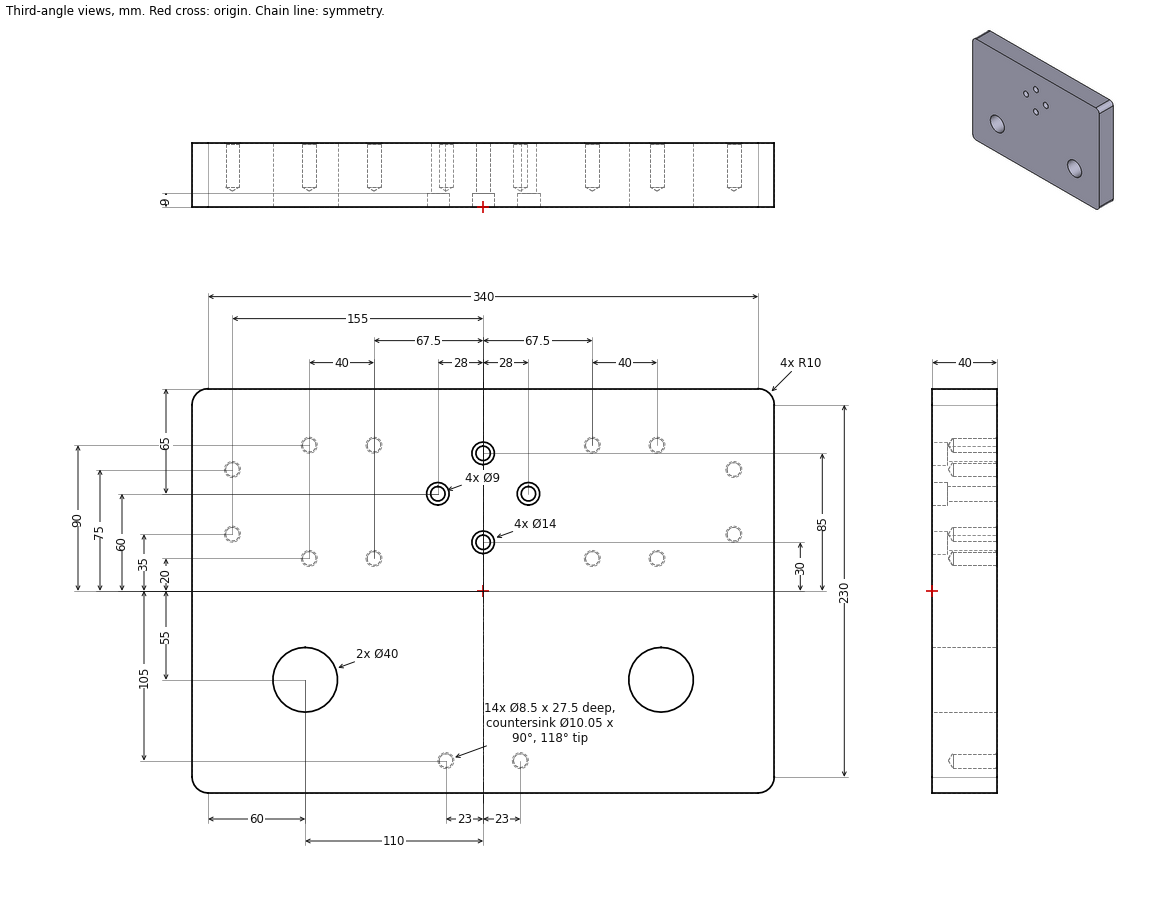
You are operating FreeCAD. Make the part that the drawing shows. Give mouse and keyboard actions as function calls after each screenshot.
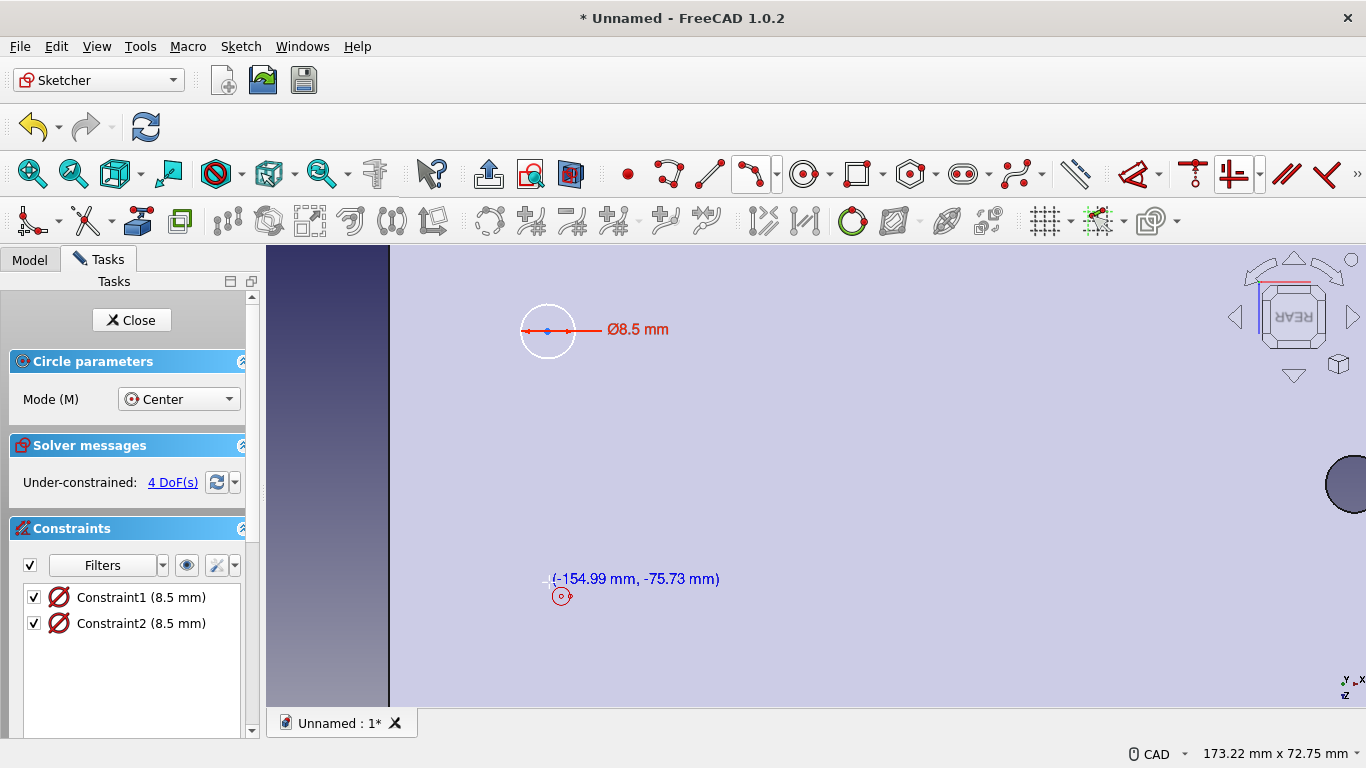
scroll(549, 582, down, 8)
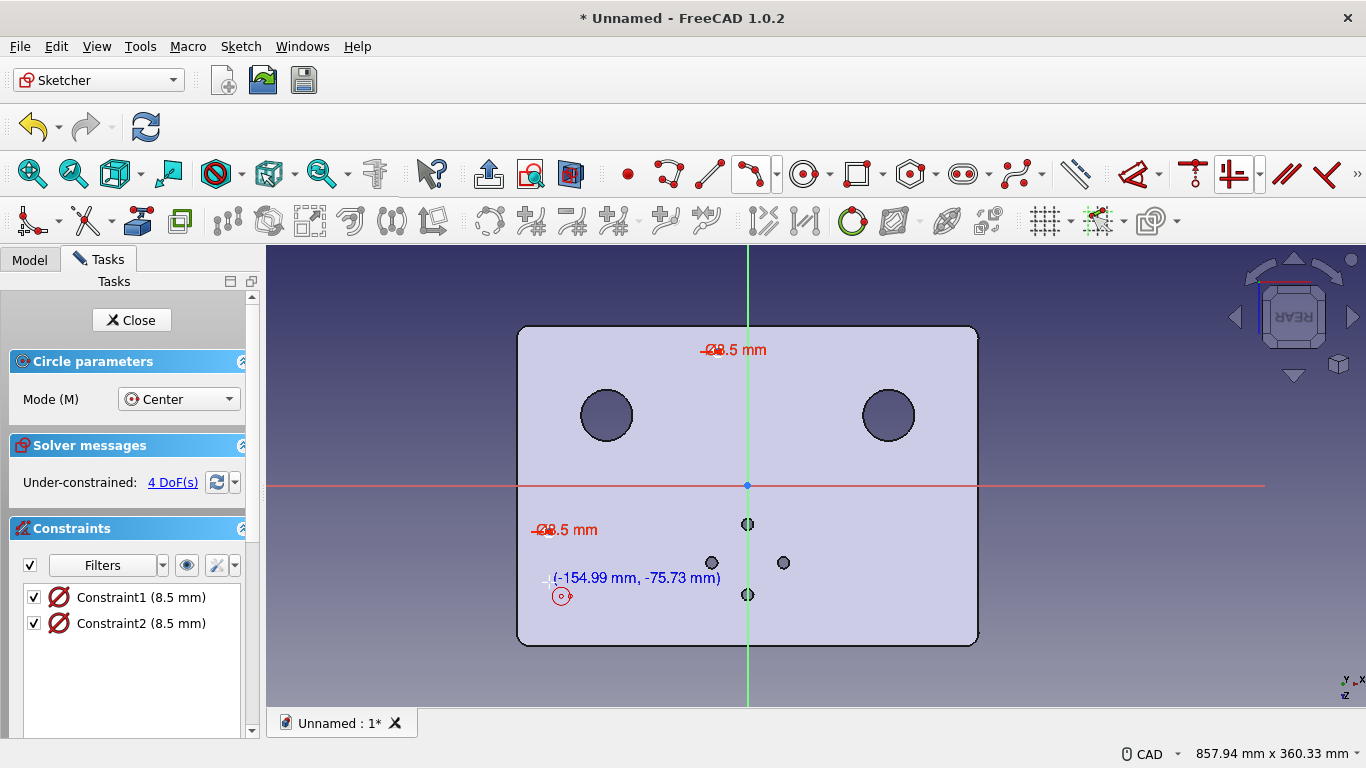
click(549, 582)
move(553, 578)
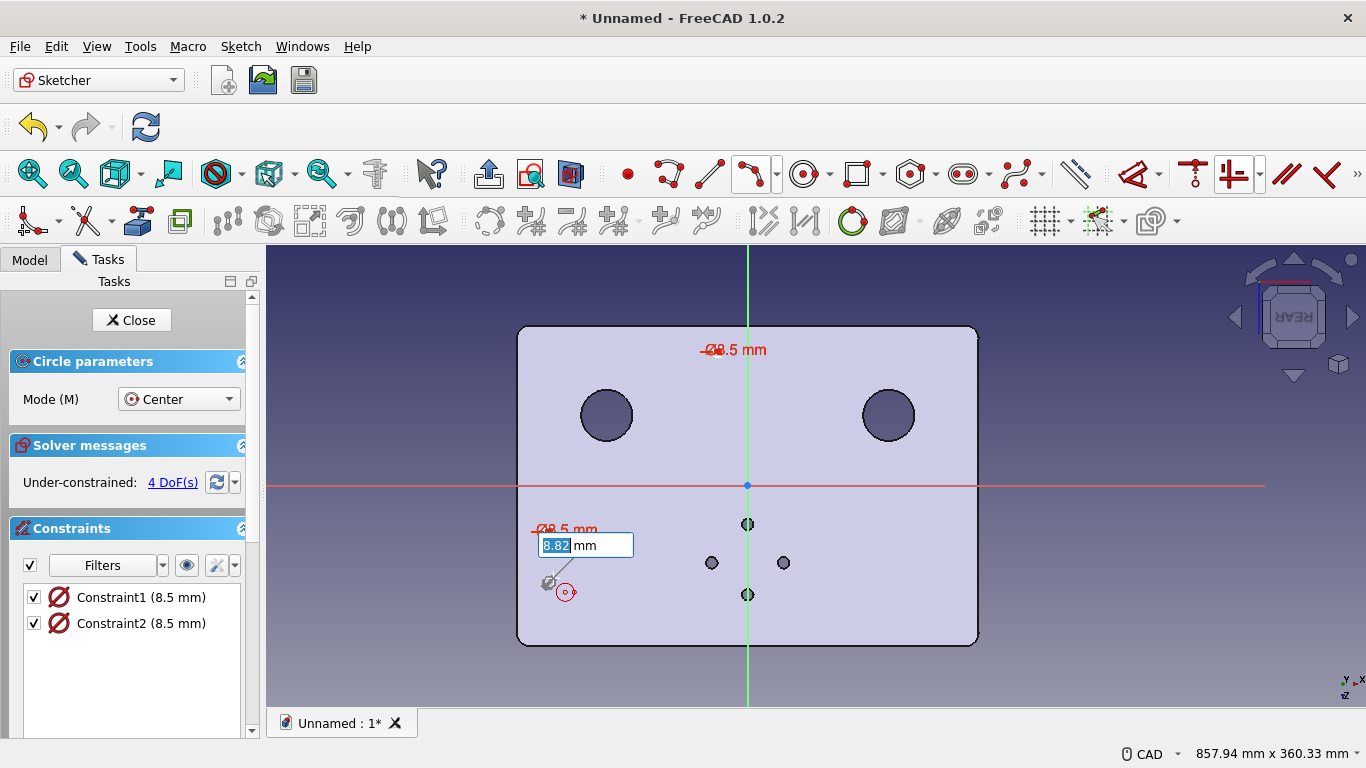
text(8.5)
key(Return)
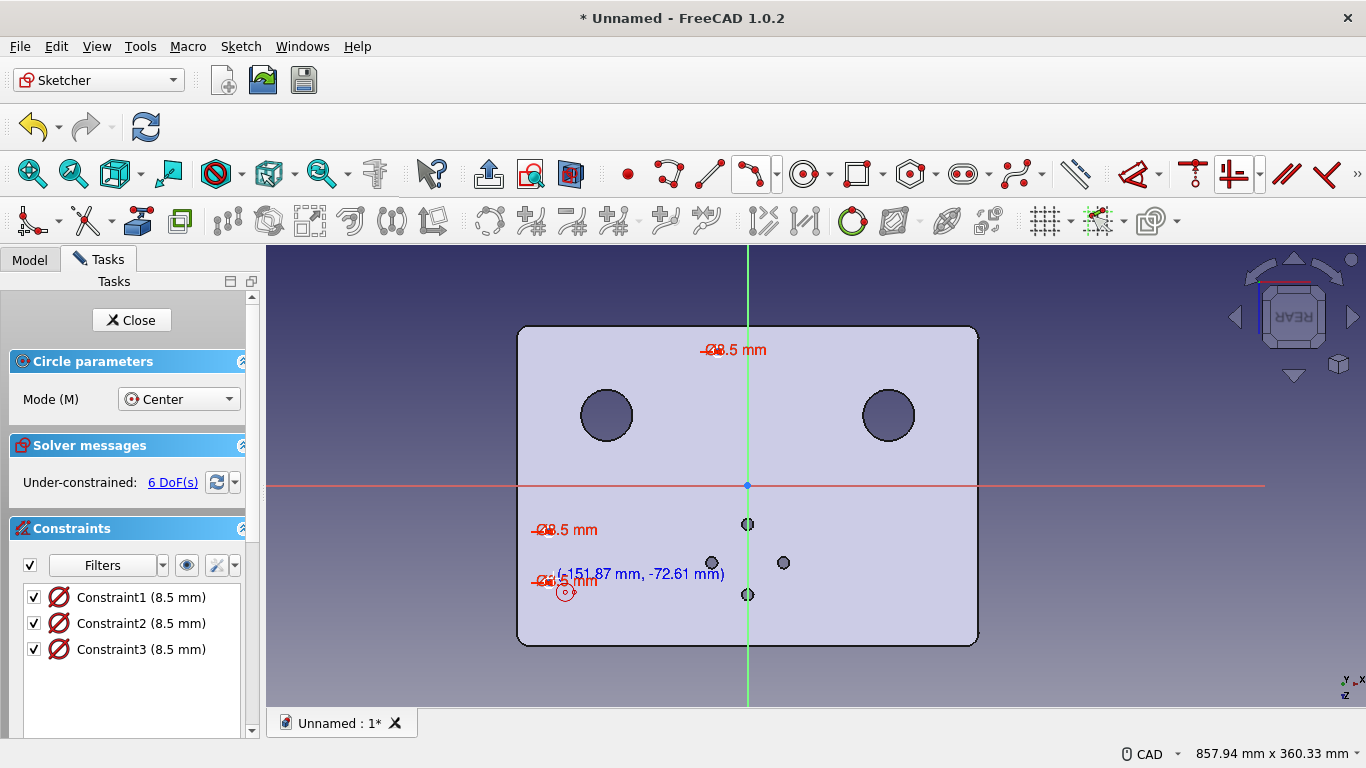
scroll(610, 512, up, 8)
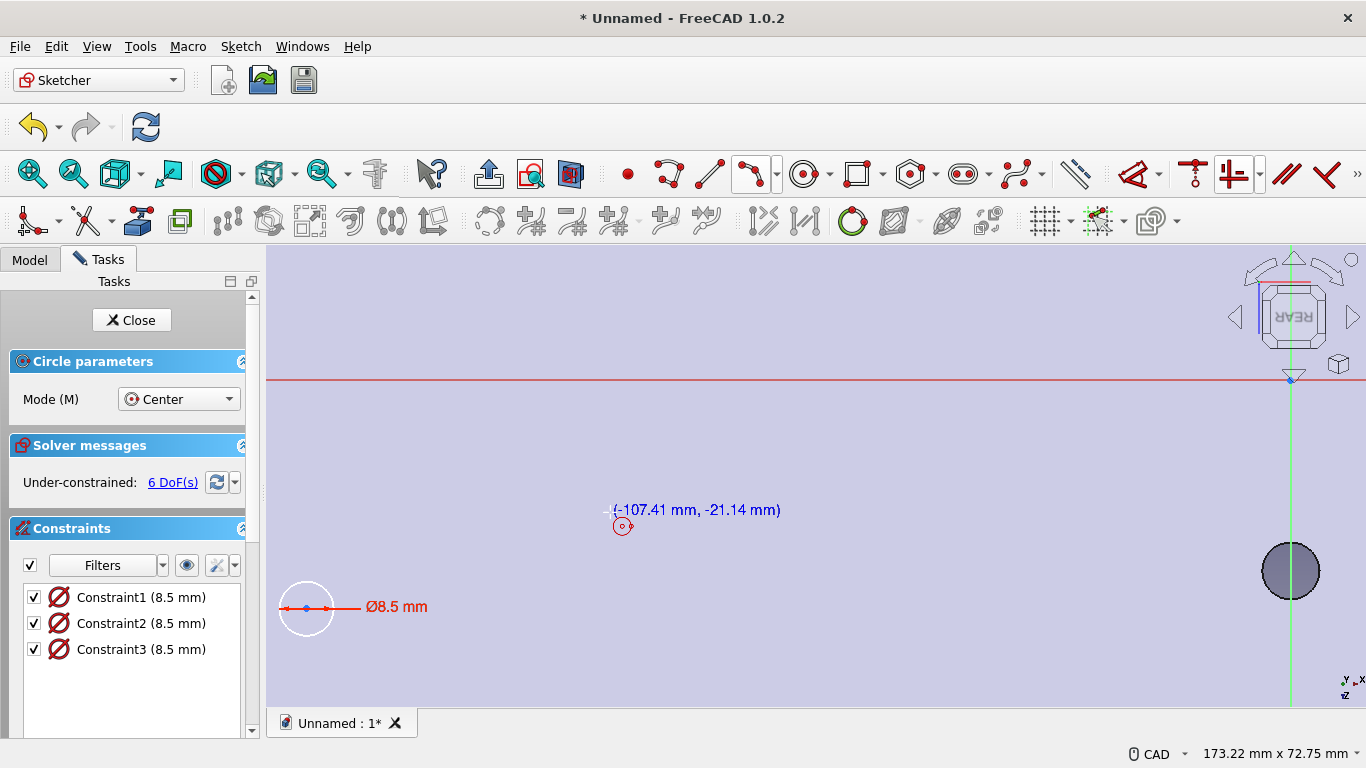
scroll(610, 512, down, 8)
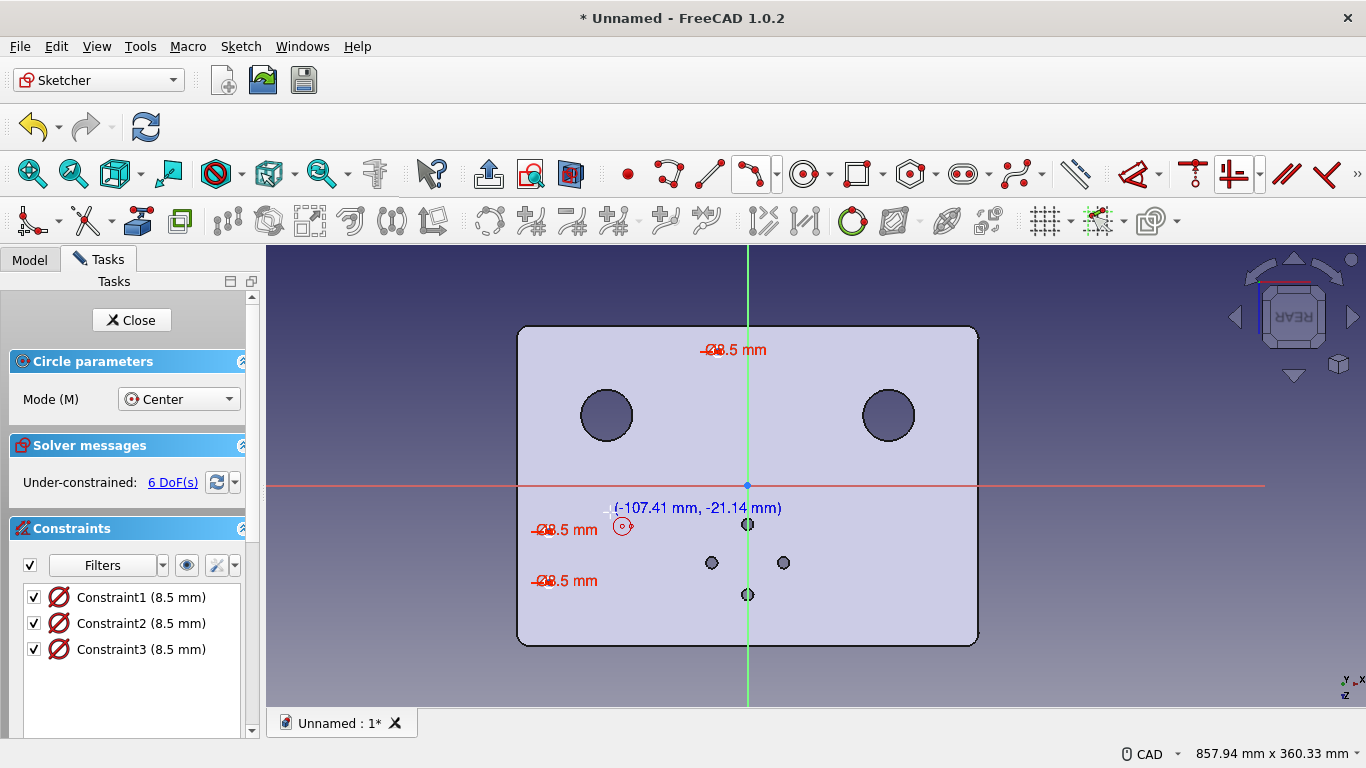
click(610, 512)
move(614, 508)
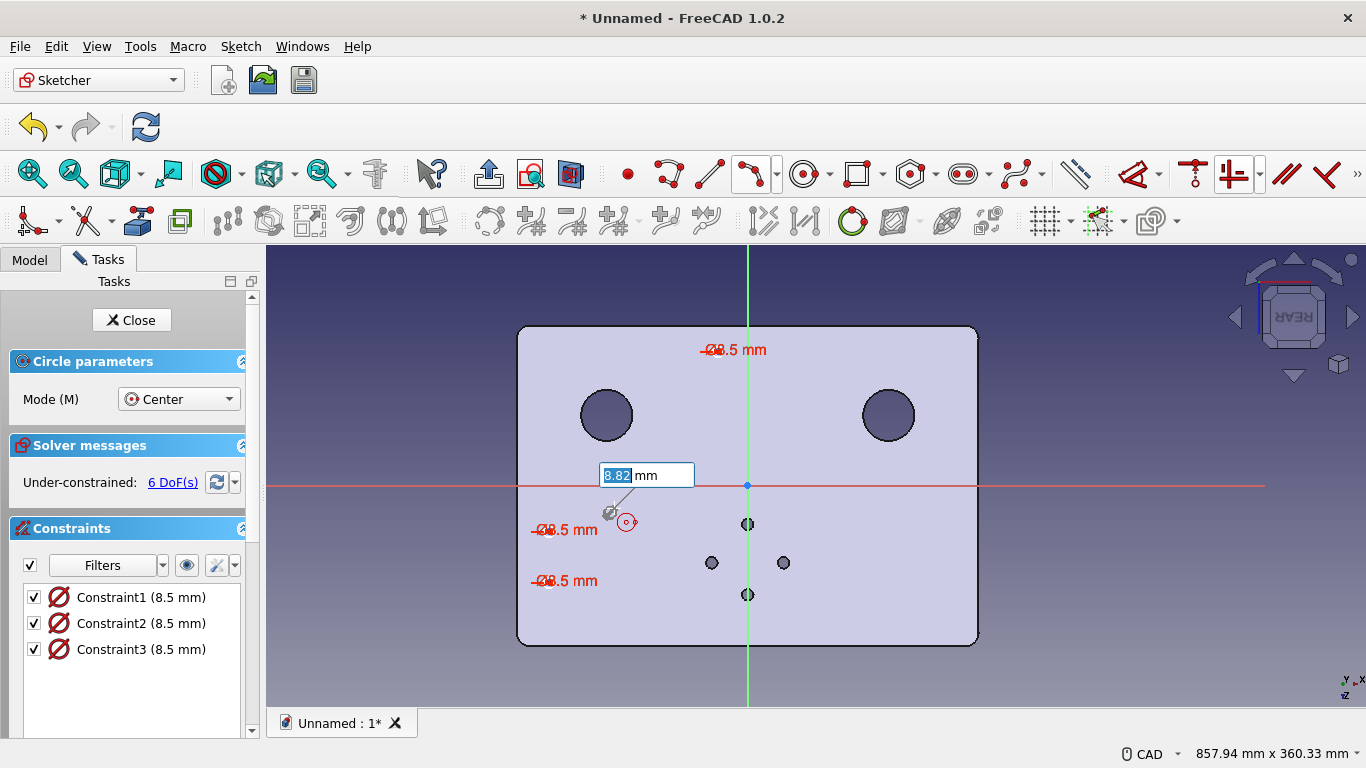
text(8.5)
key(Return)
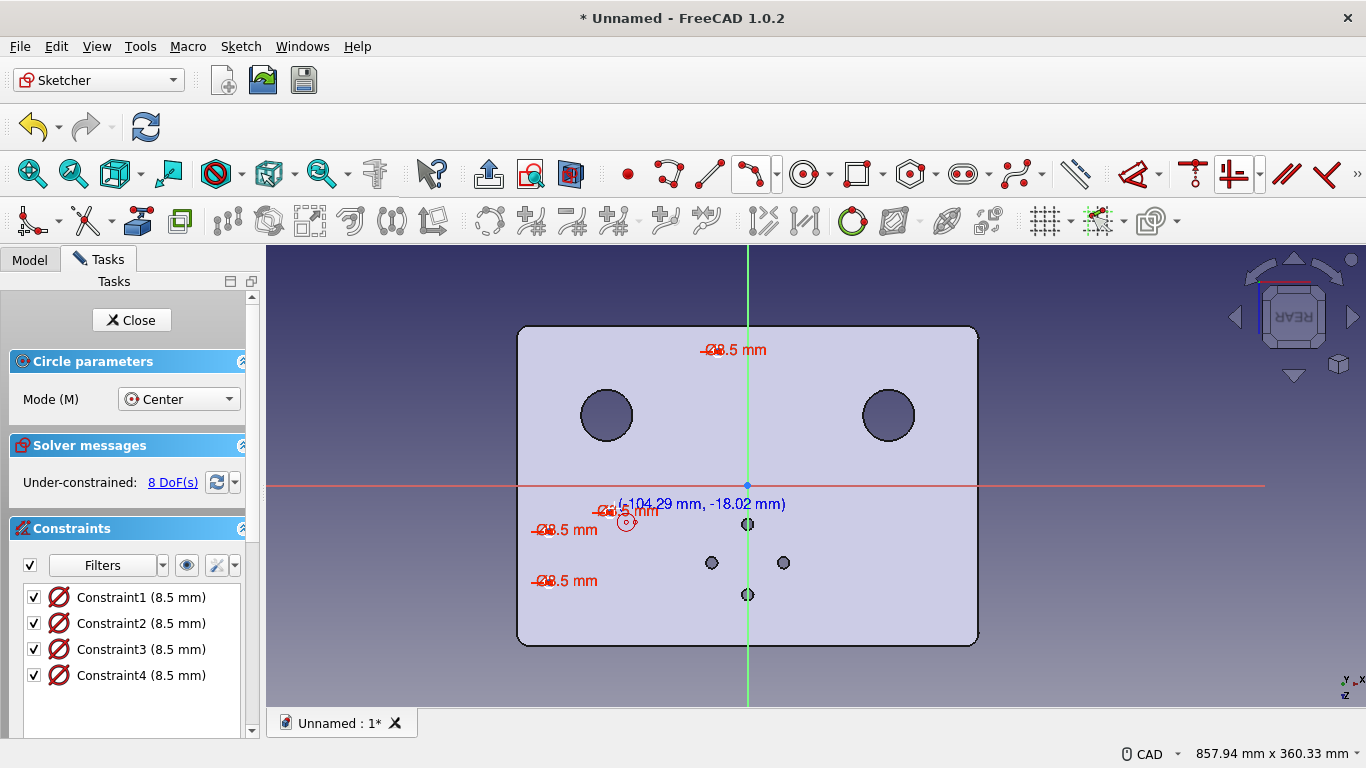
scroll(661, 512, up, 8)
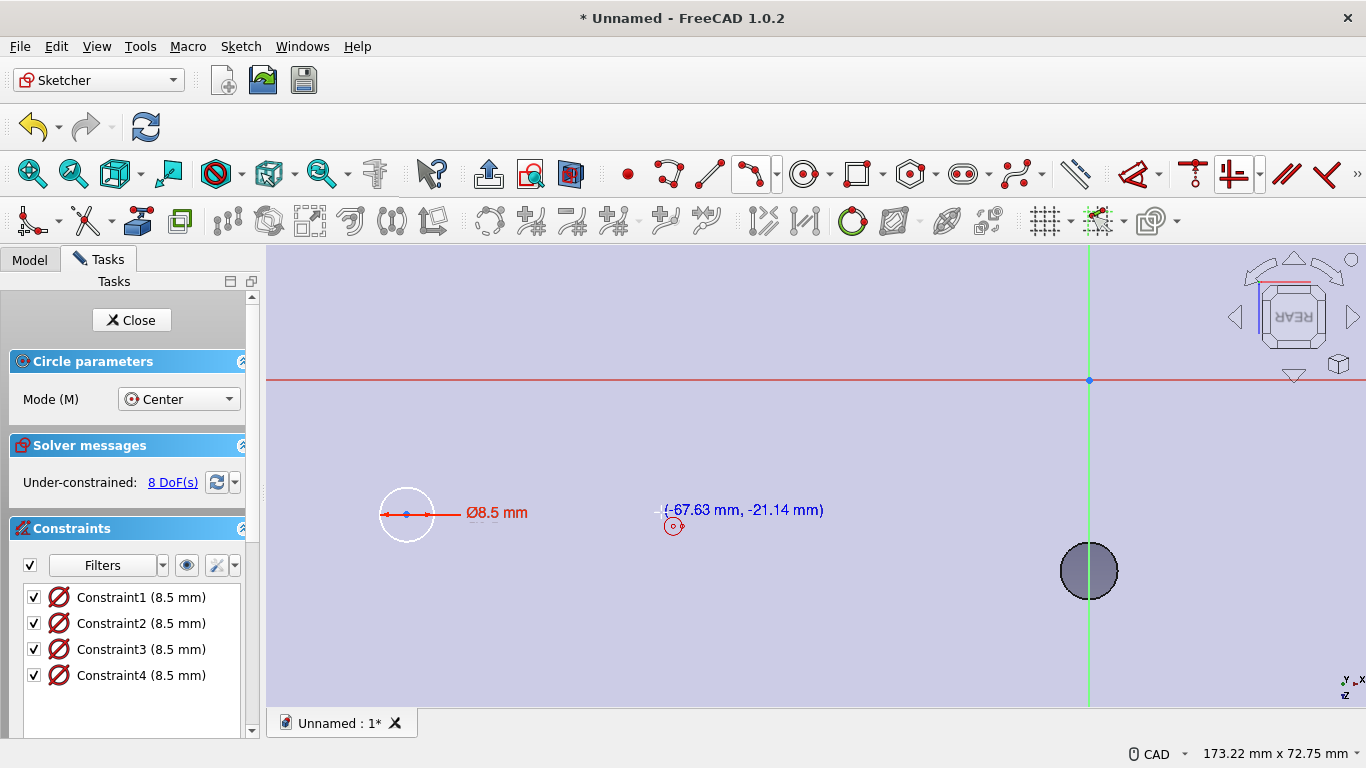
scroll(661, 512, down, 8)